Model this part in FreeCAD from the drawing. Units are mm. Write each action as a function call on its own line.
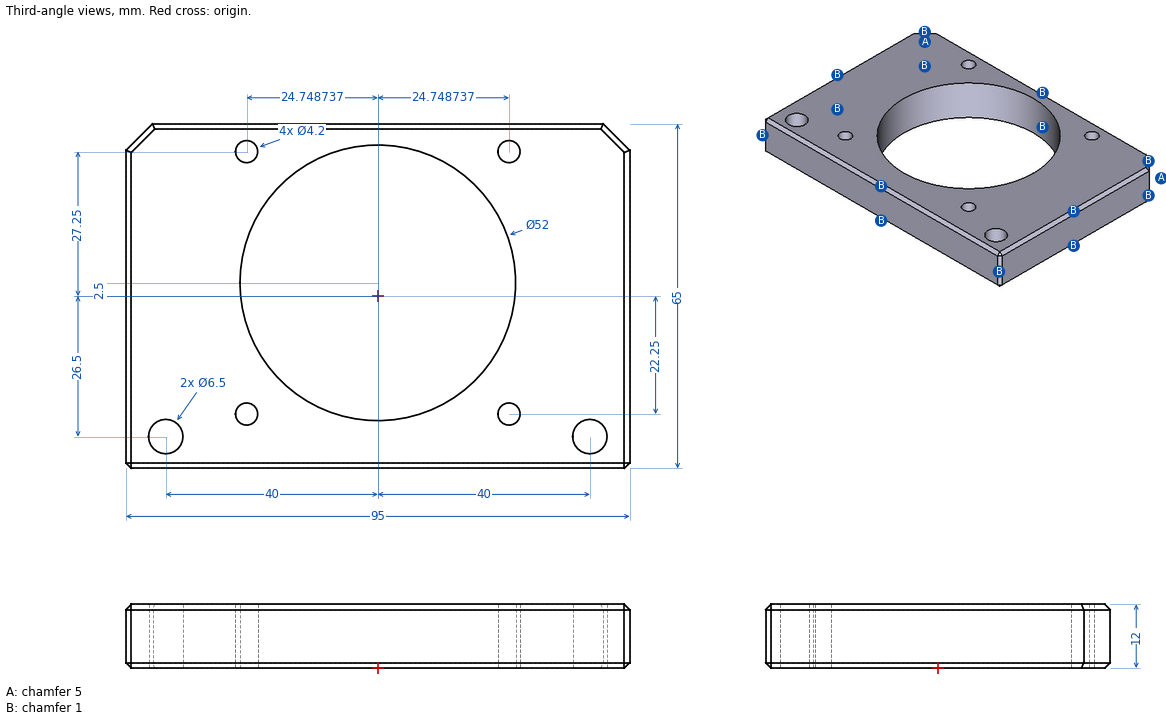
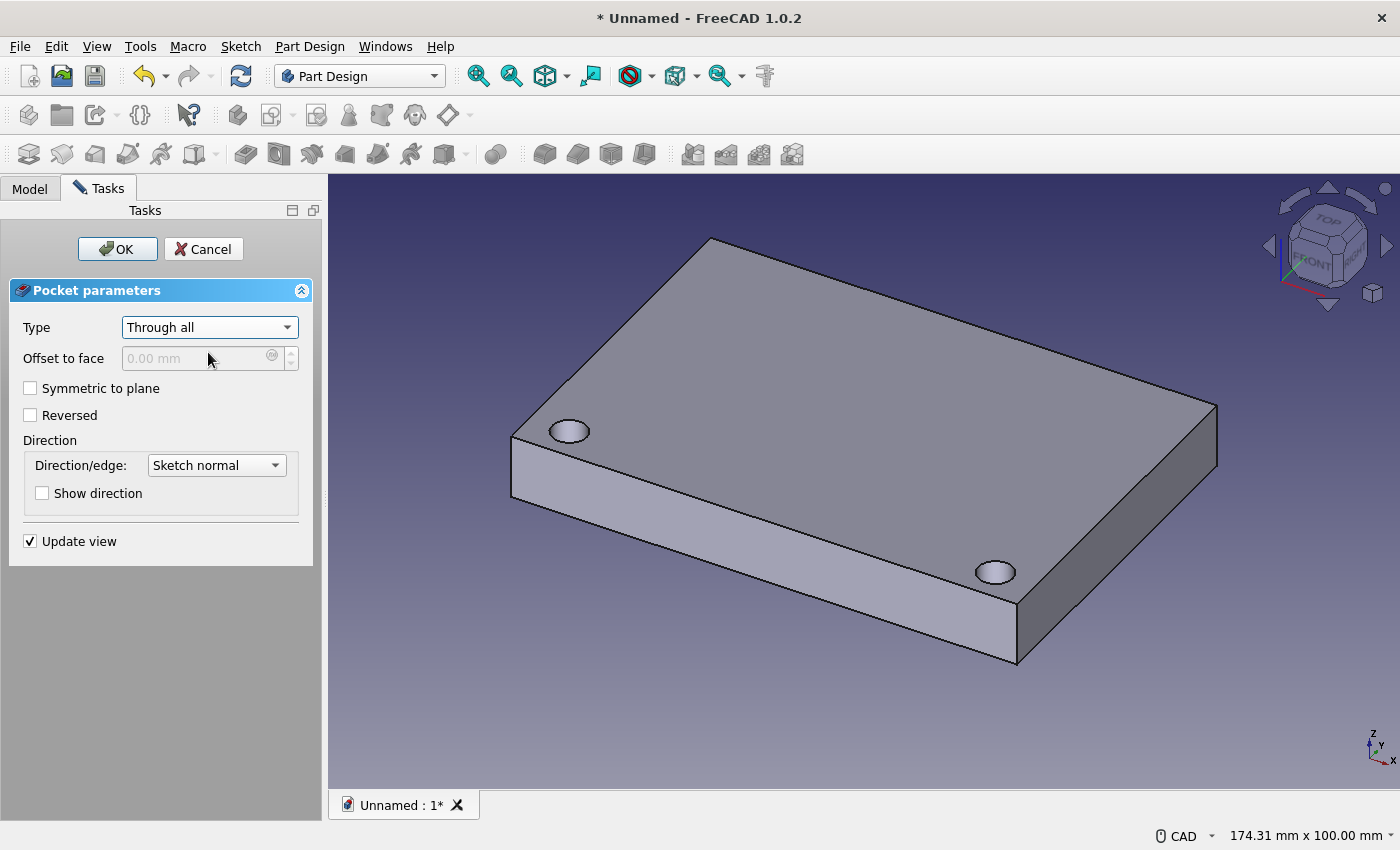
click(118, 249)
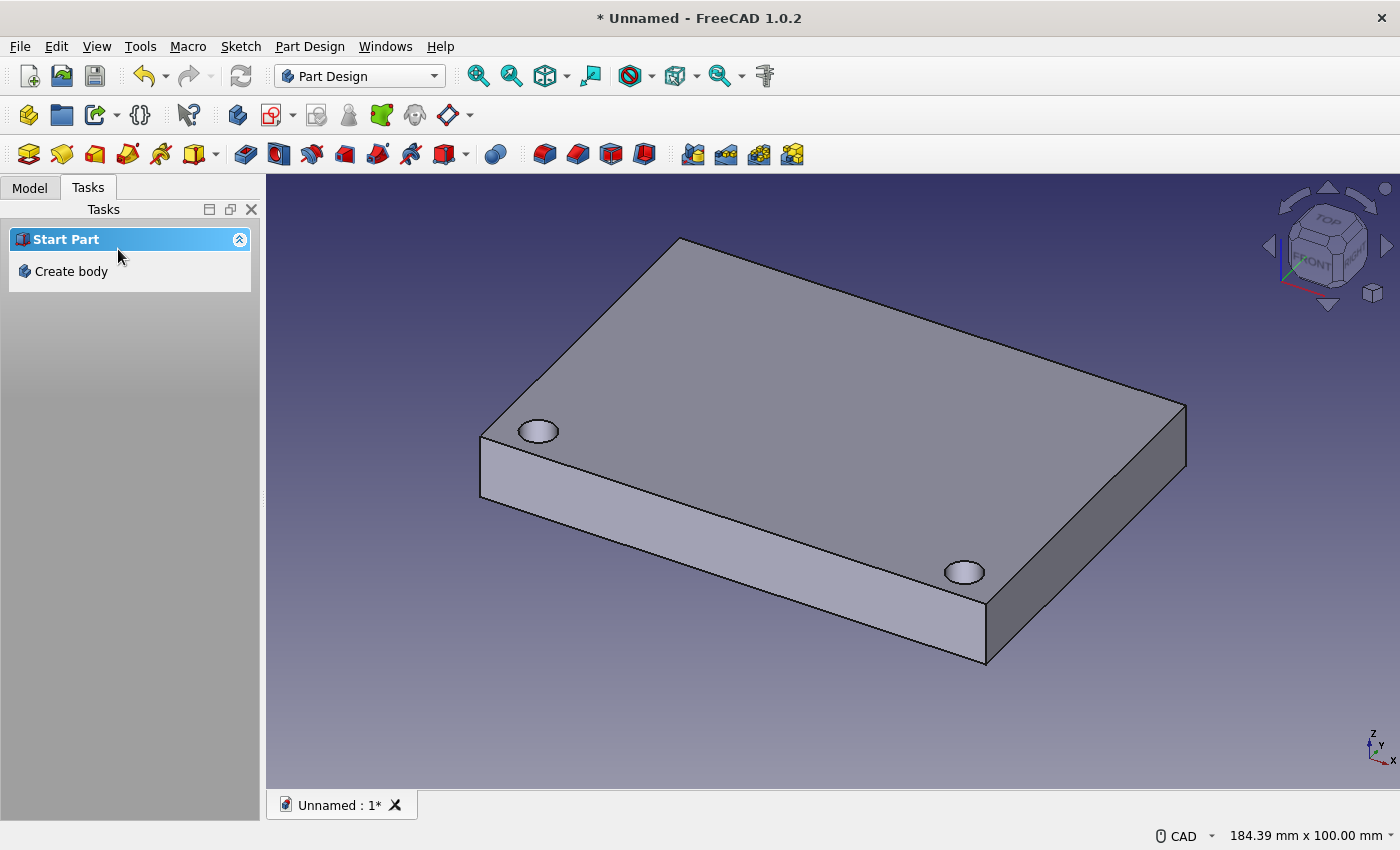
key(0)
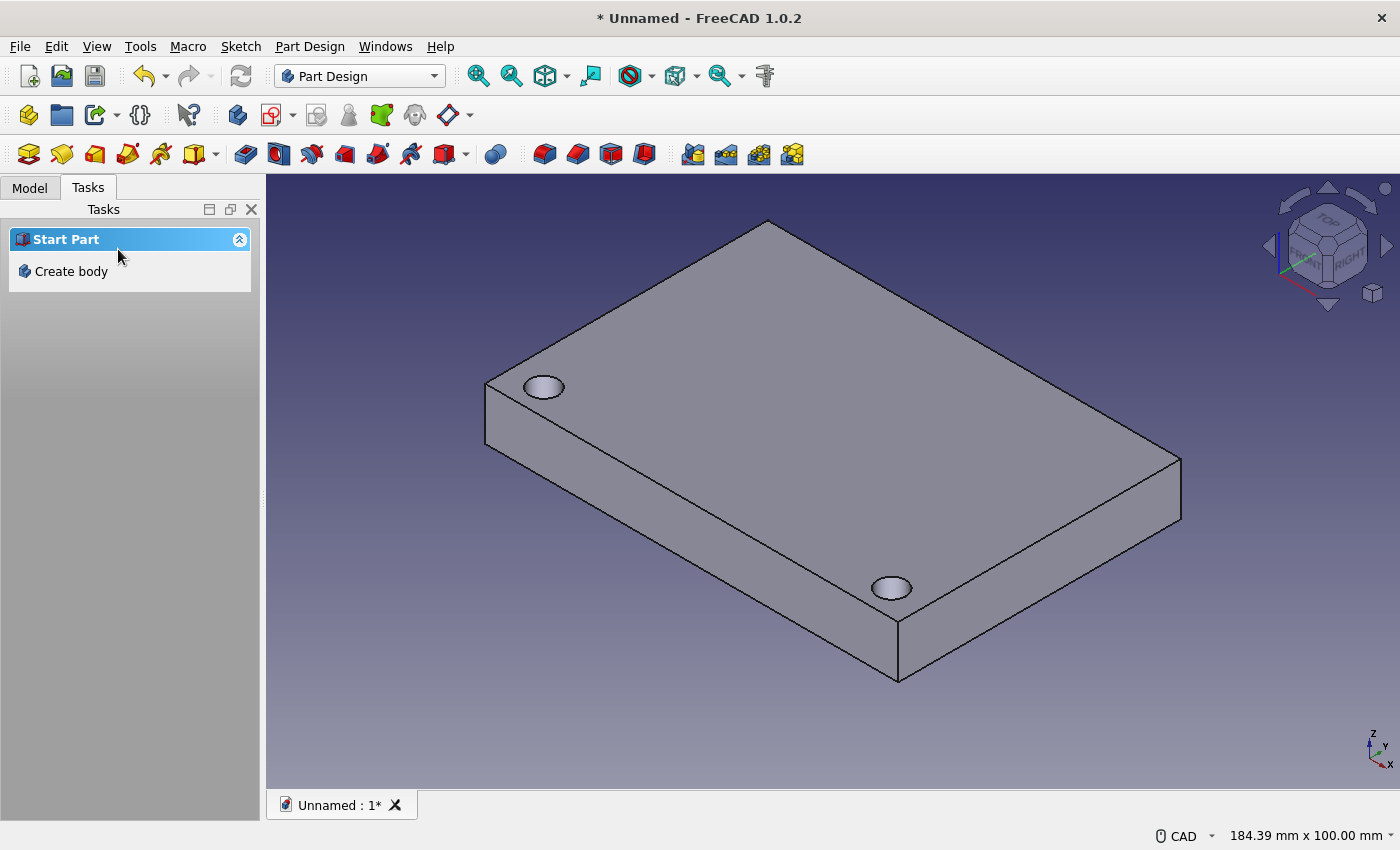
key(2)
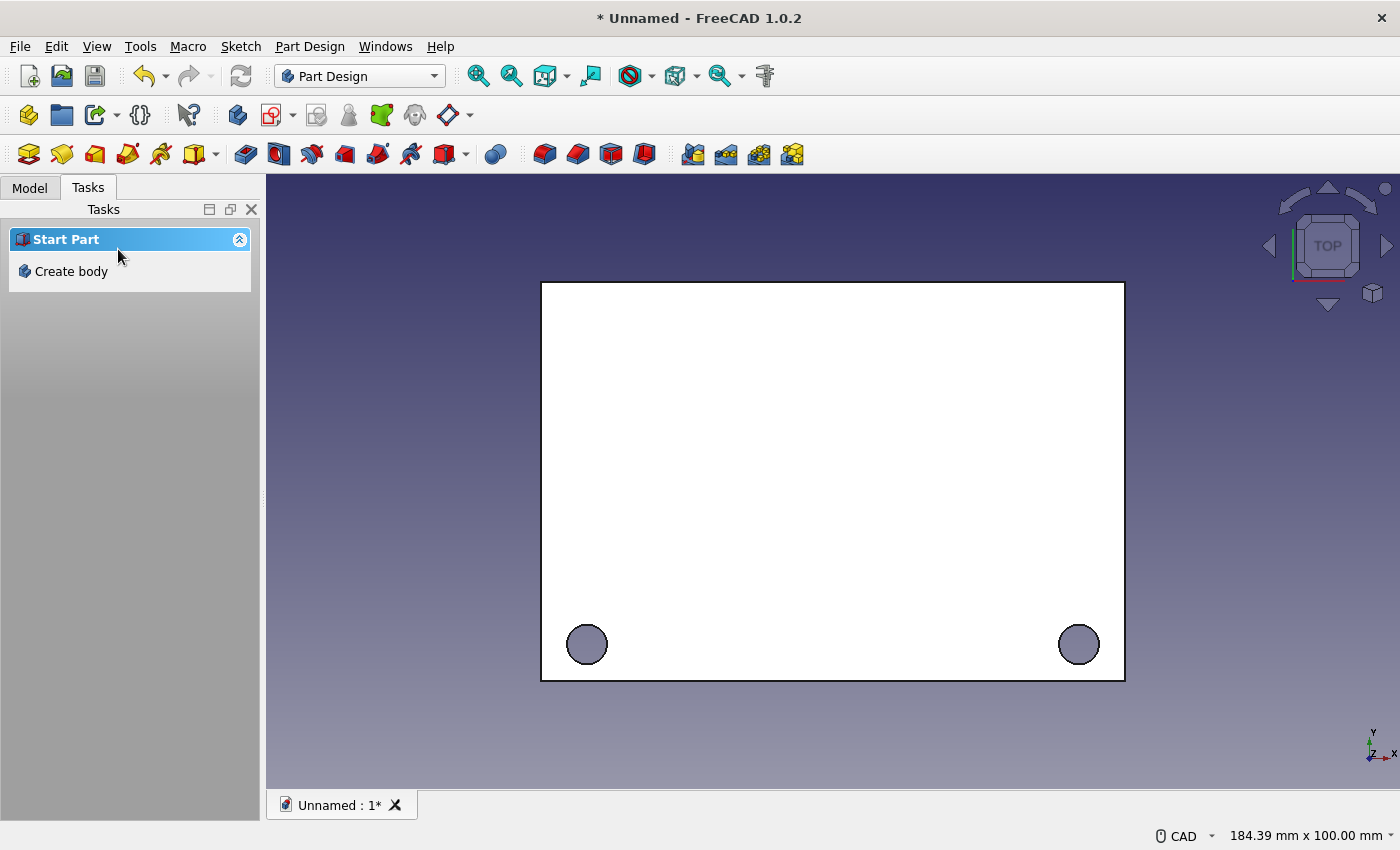
key(1)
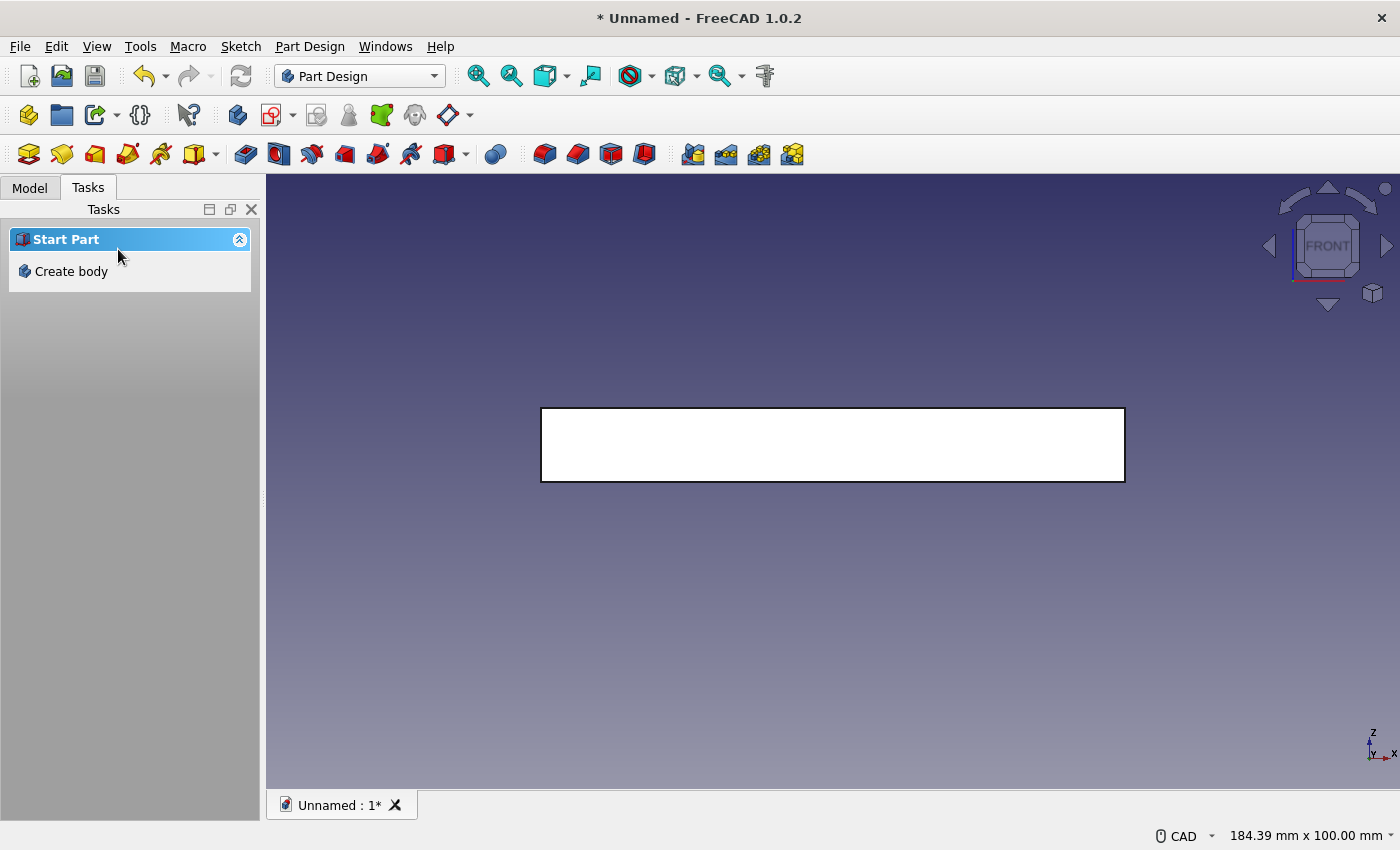
key(3)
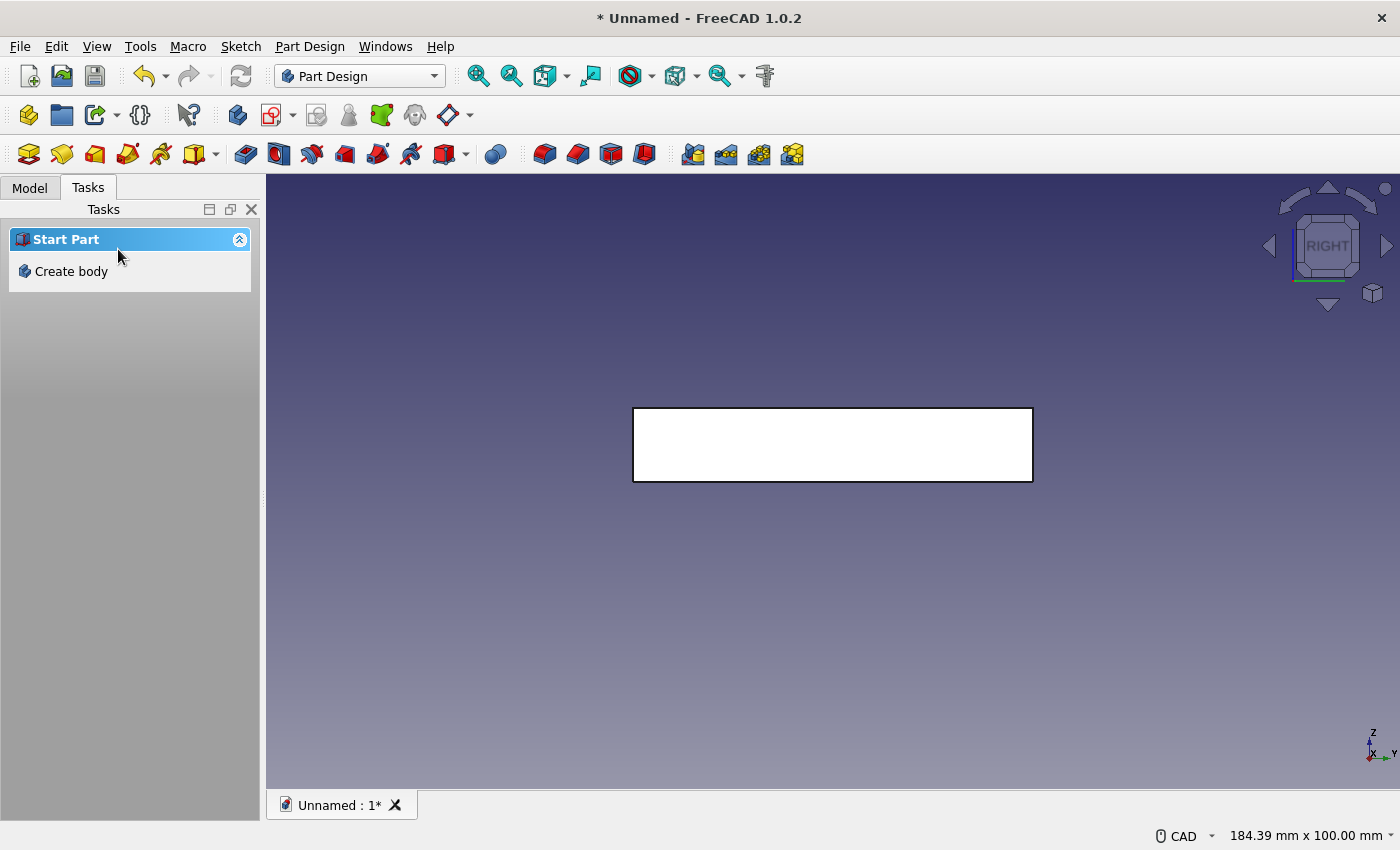
click(479, 76)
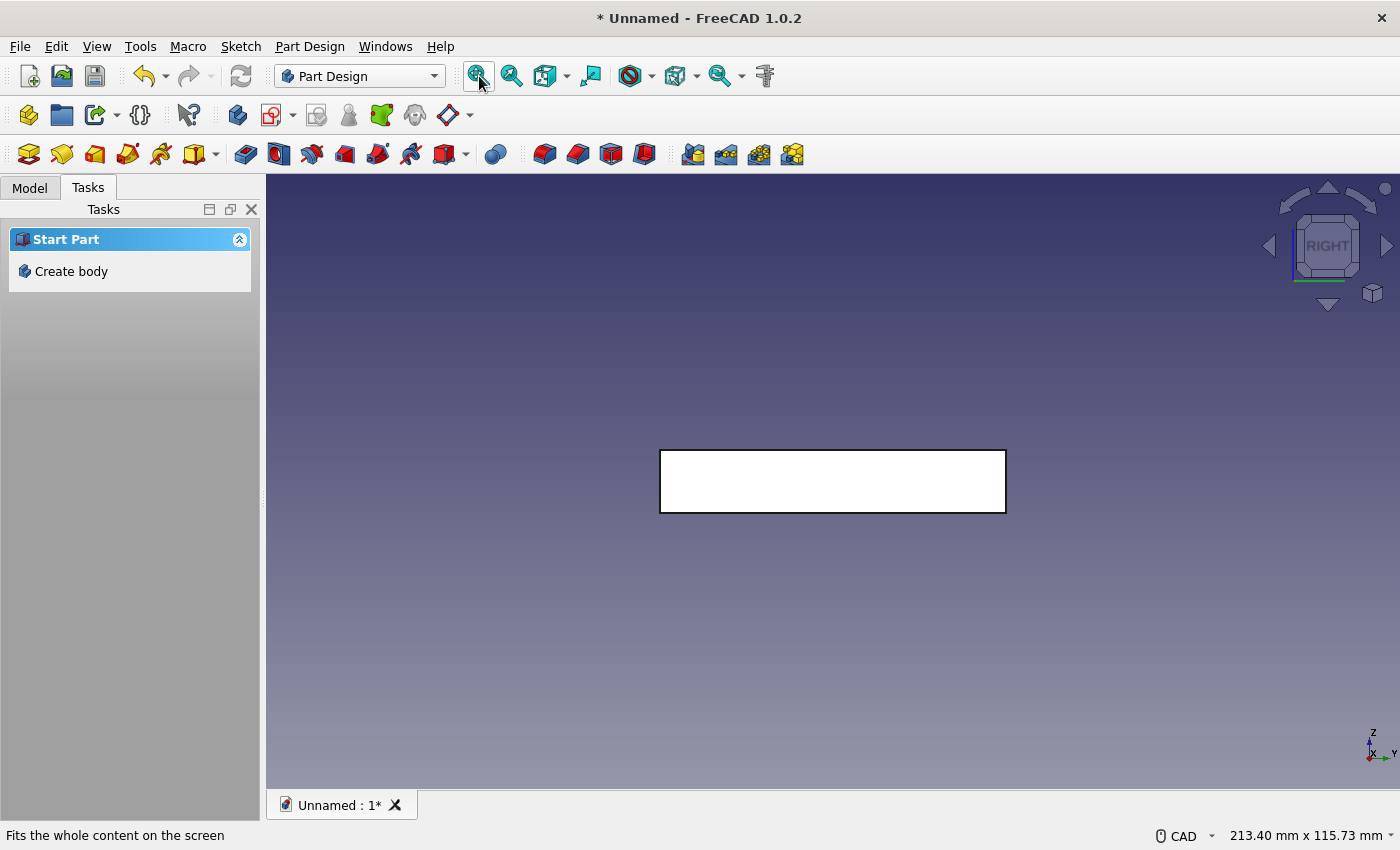
click(1006, 480)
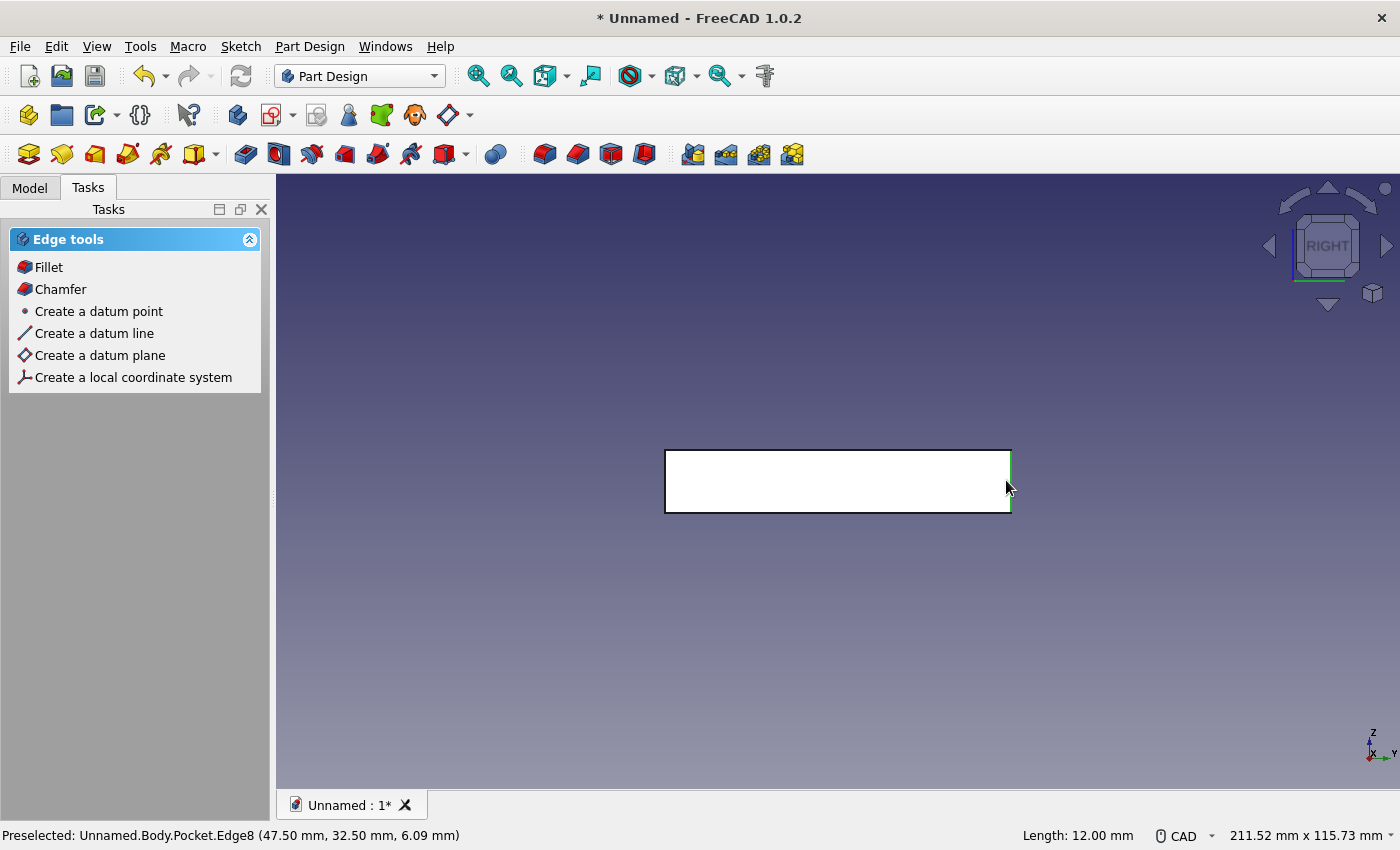
key(5)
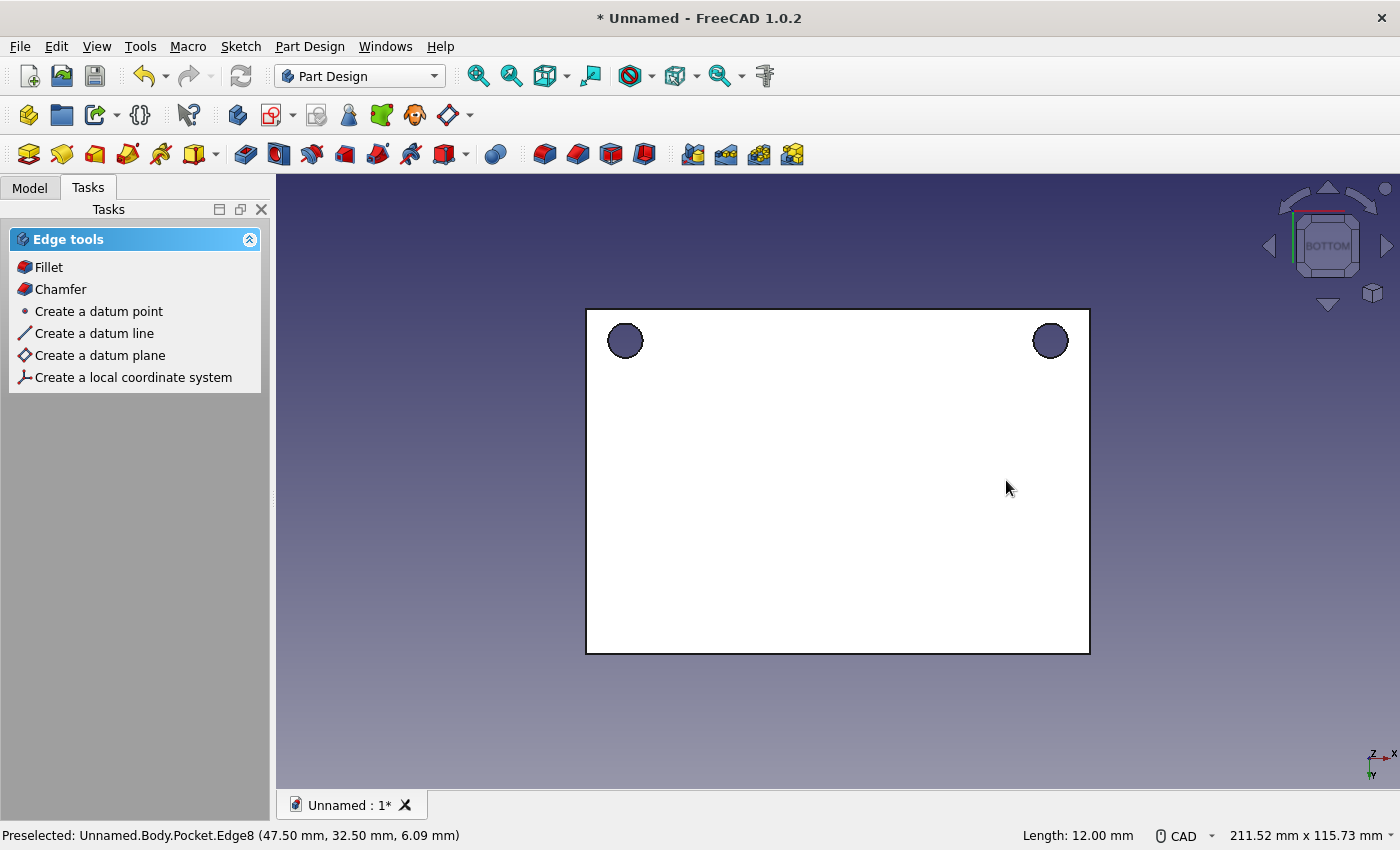
key(4)